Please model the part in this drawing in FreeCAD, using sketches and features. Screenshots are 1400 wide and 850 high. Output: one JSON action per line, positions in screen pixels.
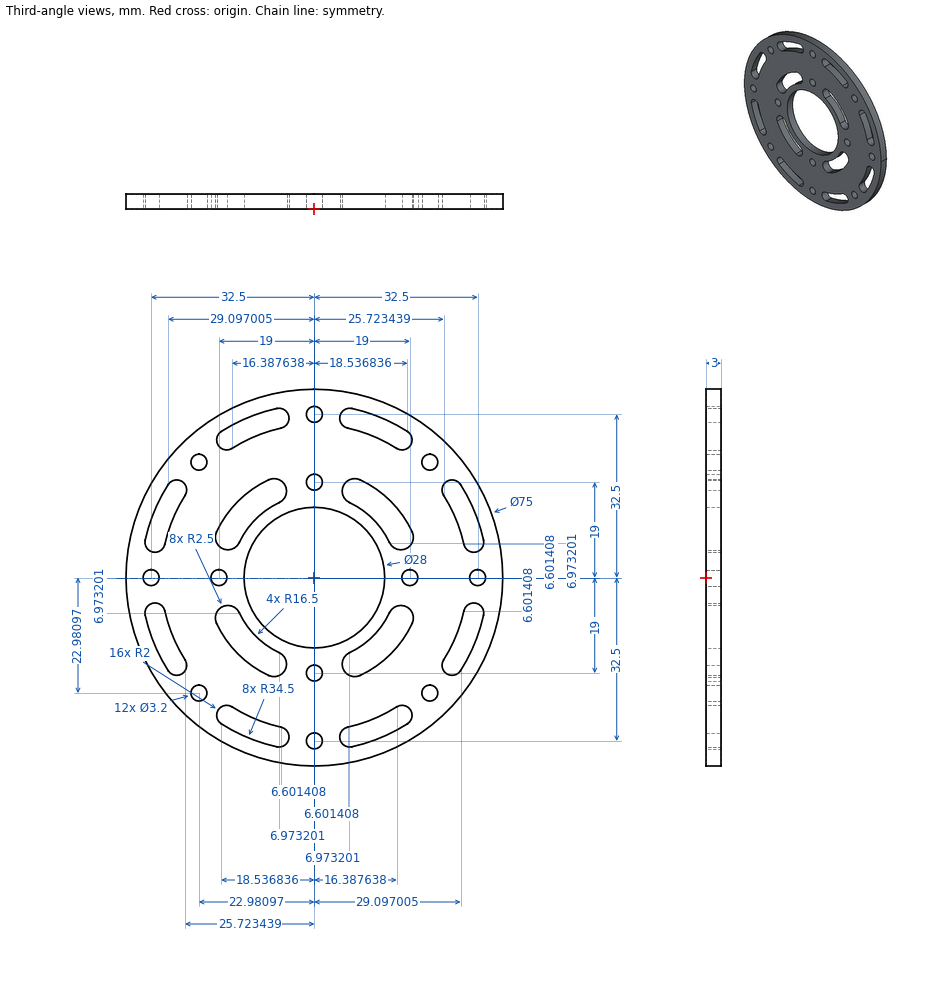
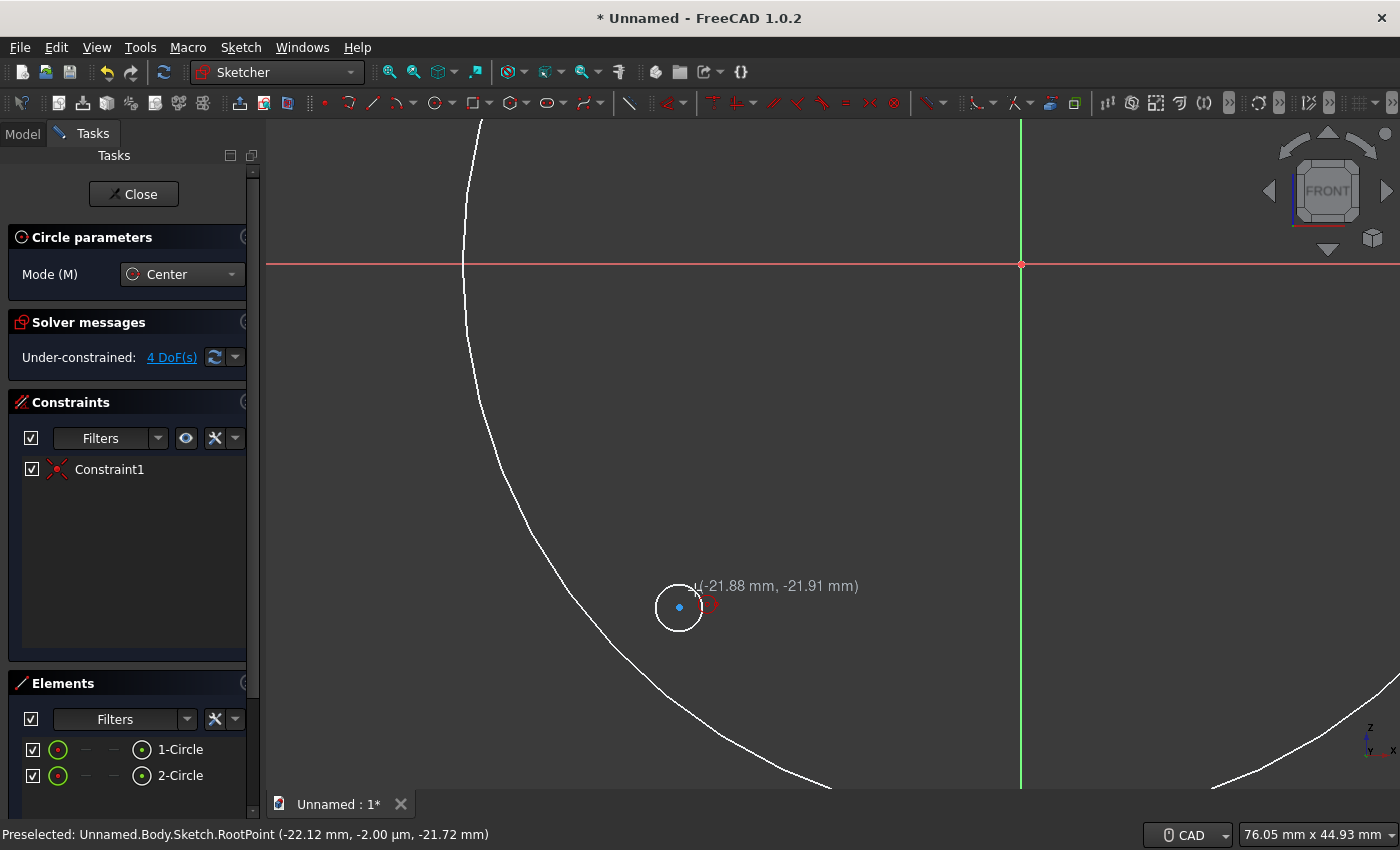
{"action": "left_click", "coordinate": [1021, 749]}
{"action": "left_click", "coordinate": [1038, 732]}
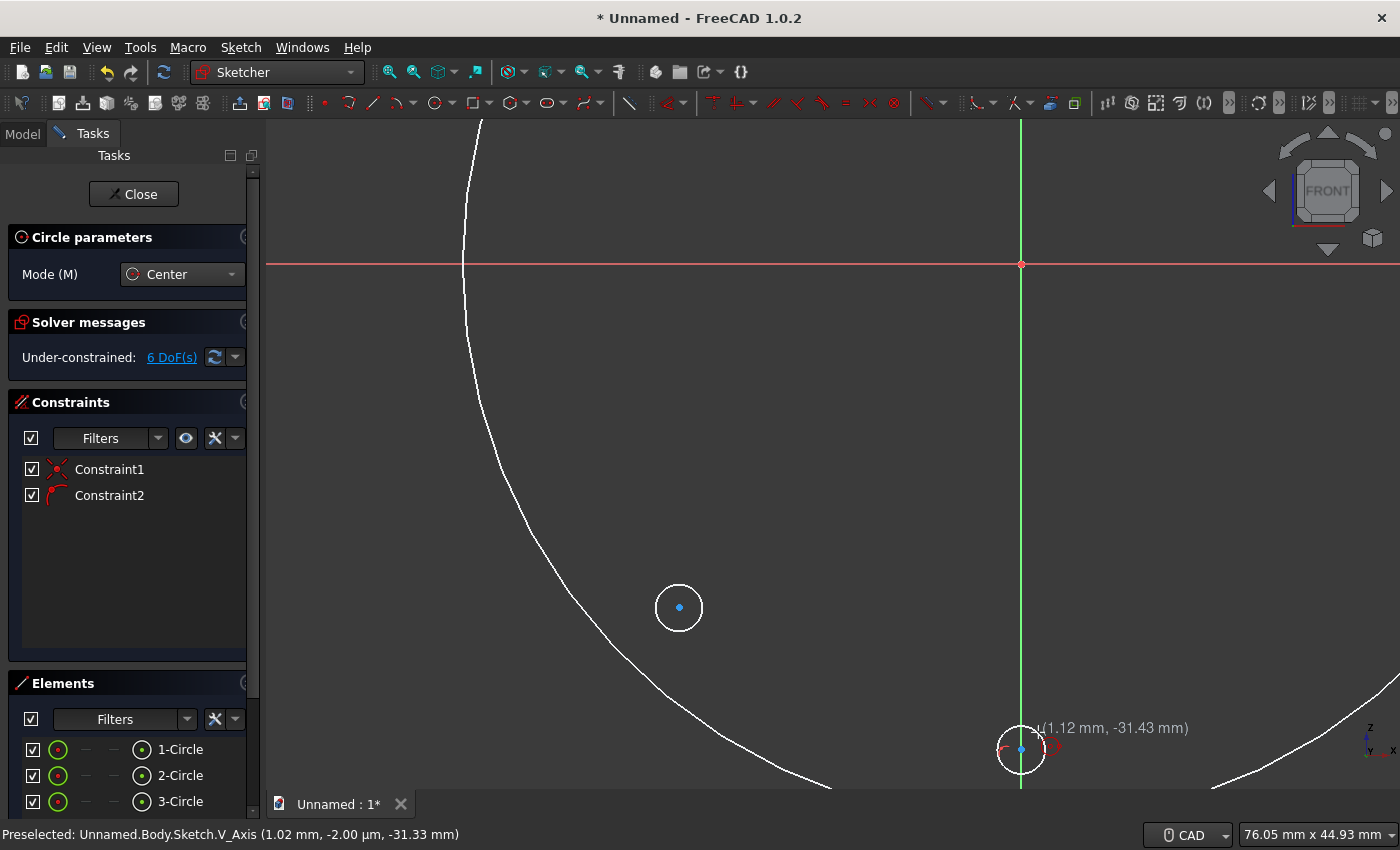
{"action": "left_click", "coordinate": [1021, 548]}
{"action": "left_click", "coordinate": [1038, 531]}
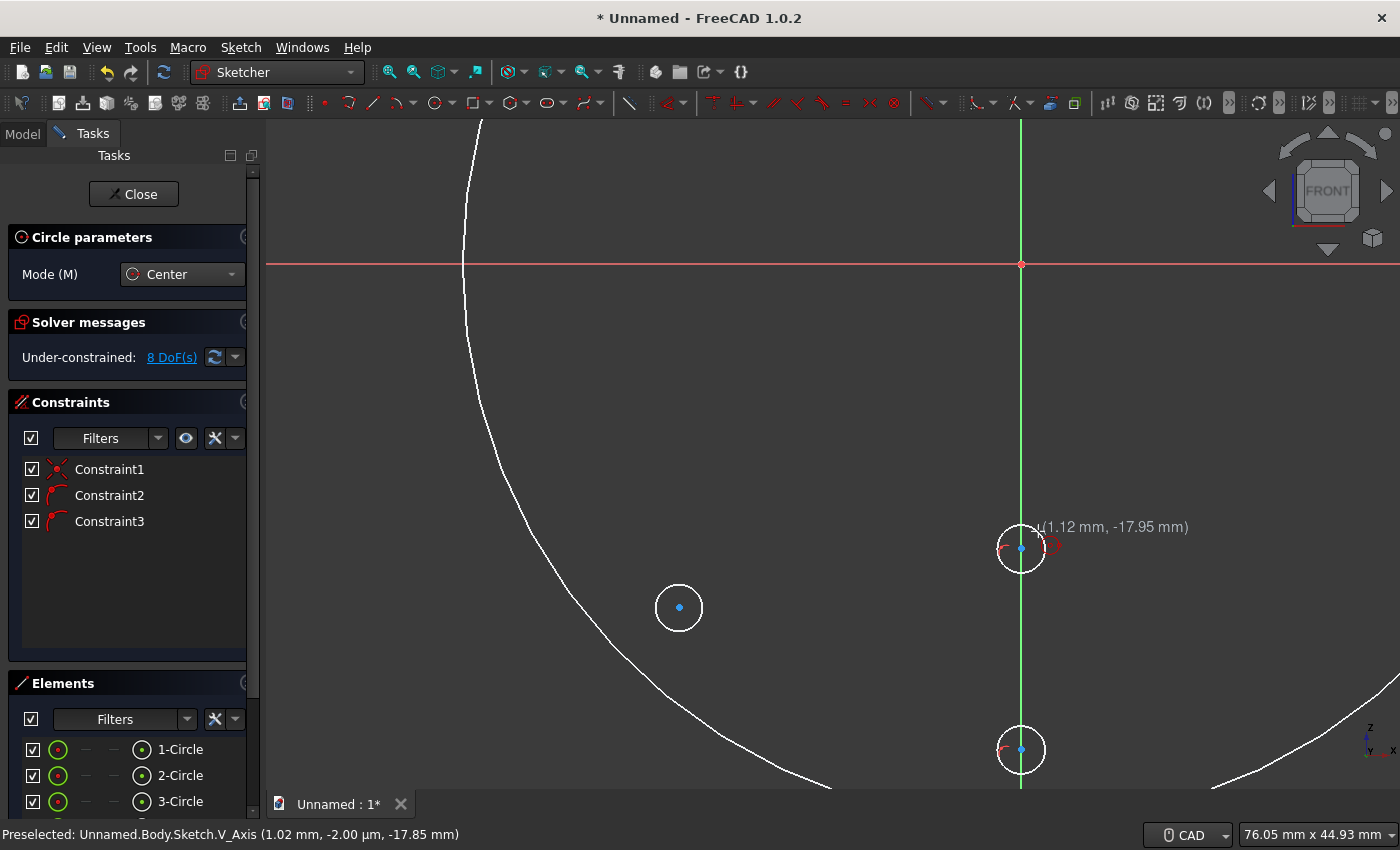
{"action": "left_click", "coordinate": [537, 264]}
{"action": "left_click", "coordinate": [554, 248]}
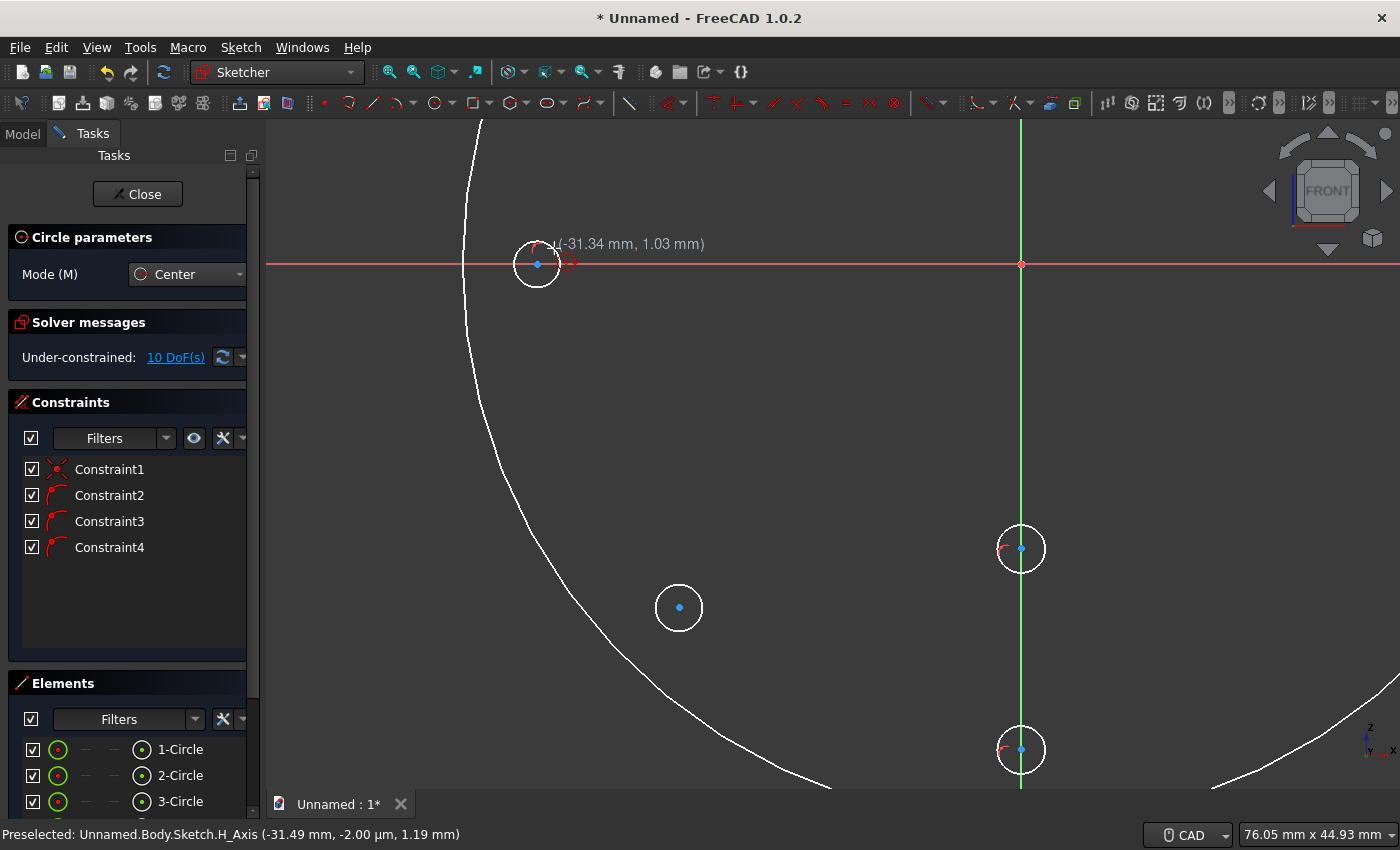
{"action": "left_click", "coordinate": [738, 264]}
{"action": "left_click", "coordinate": [755, 248]}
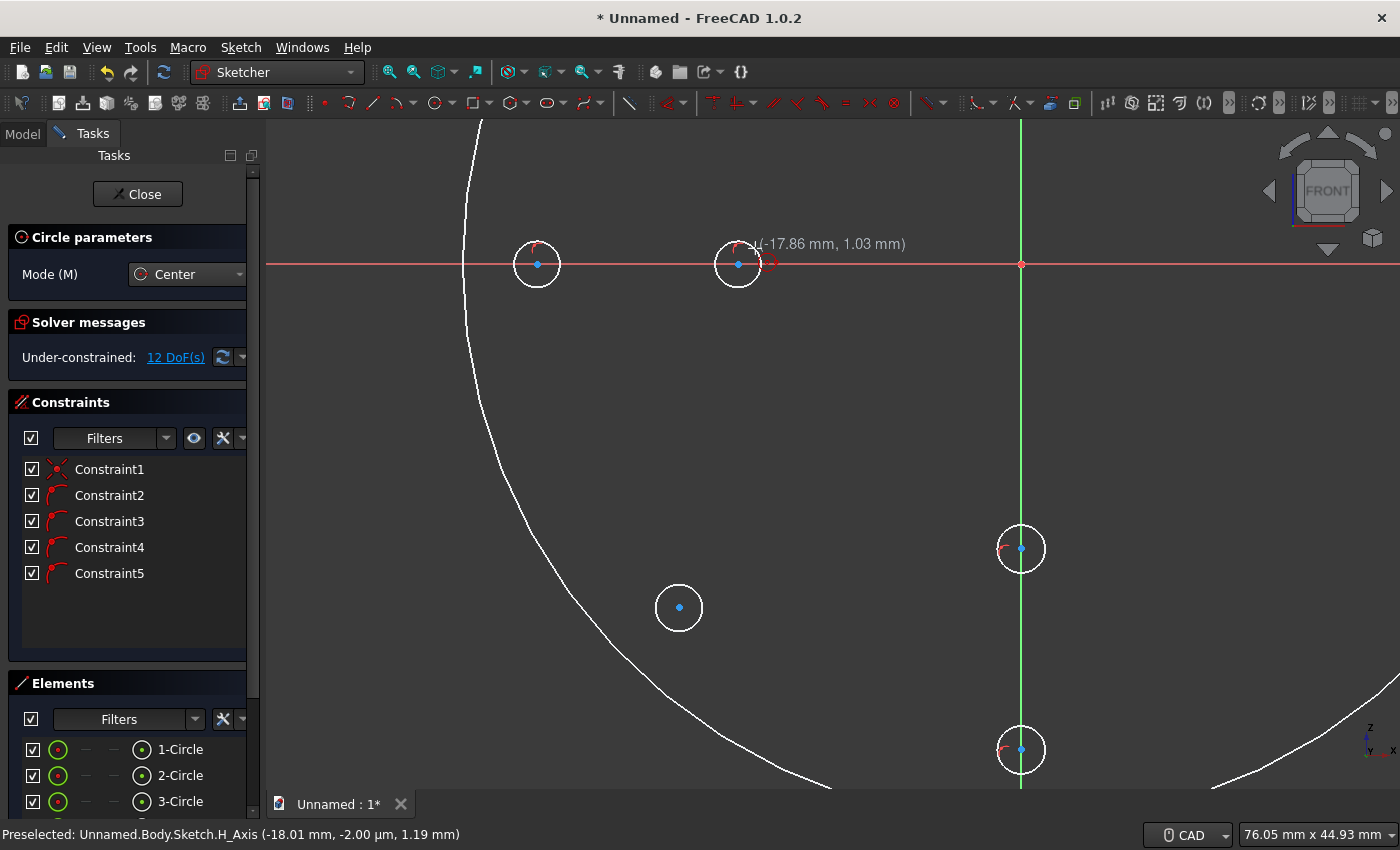
{"action": "scroll", "coordinate": [615, 564], "scroll_direction": "down", "scroll_amount": 5}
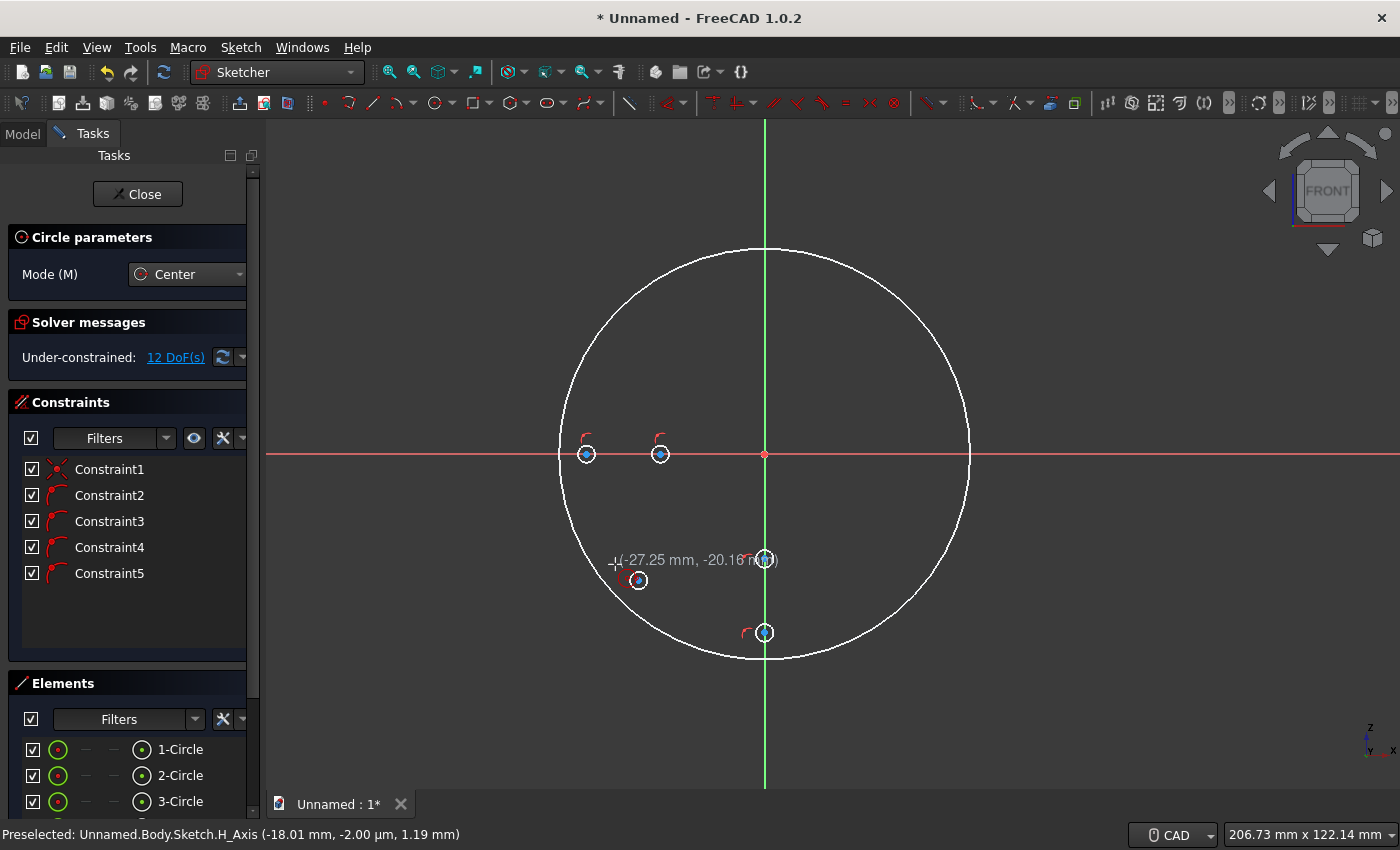
{"action": "scroll", "coordinate": [639, 328], "scroll_direction": "up", "scroll_amount": 5}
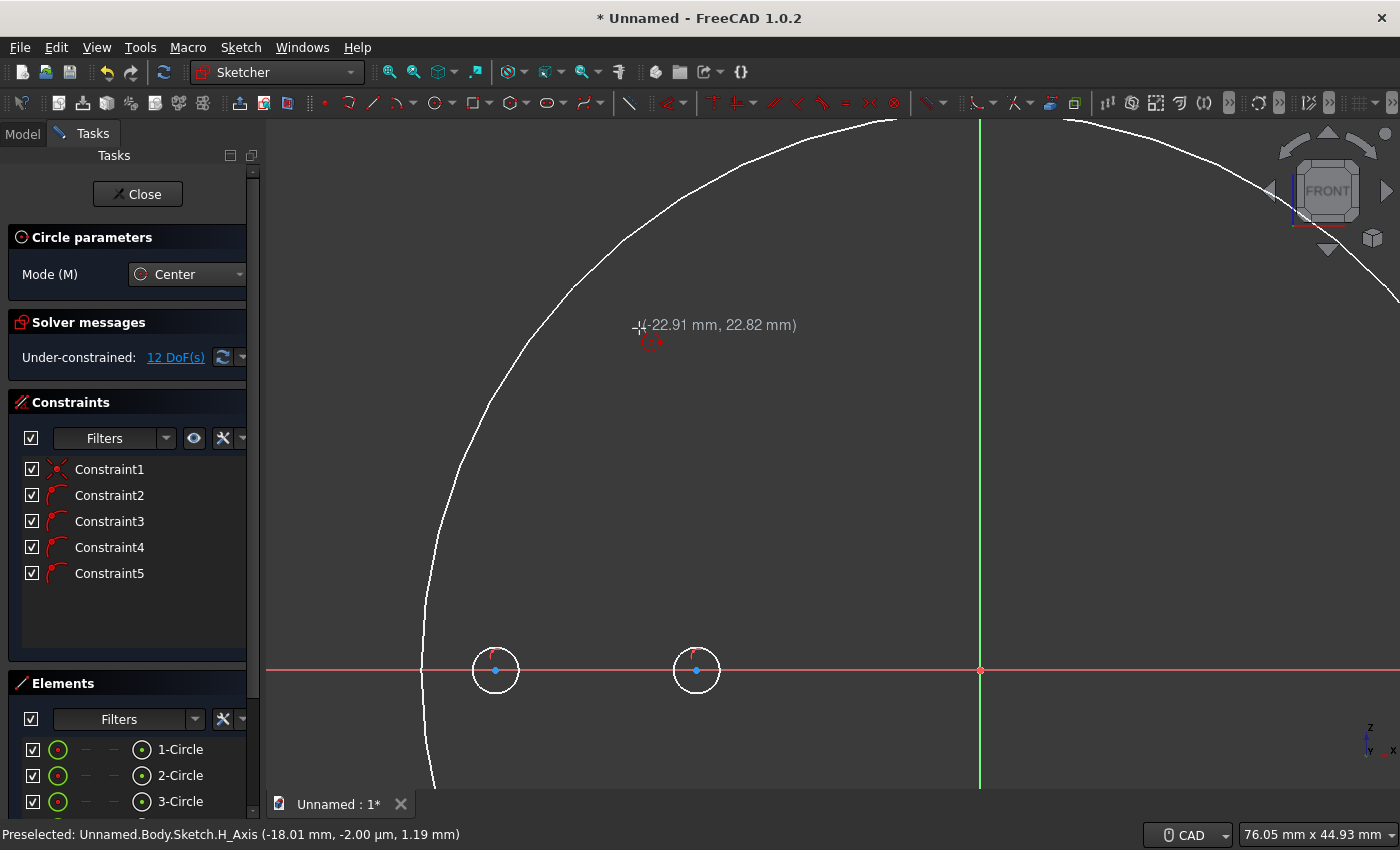
{"action": "left_click", "coordinate": [637, 328]}
{"action": "left_click", "coordinate": [654, 311]}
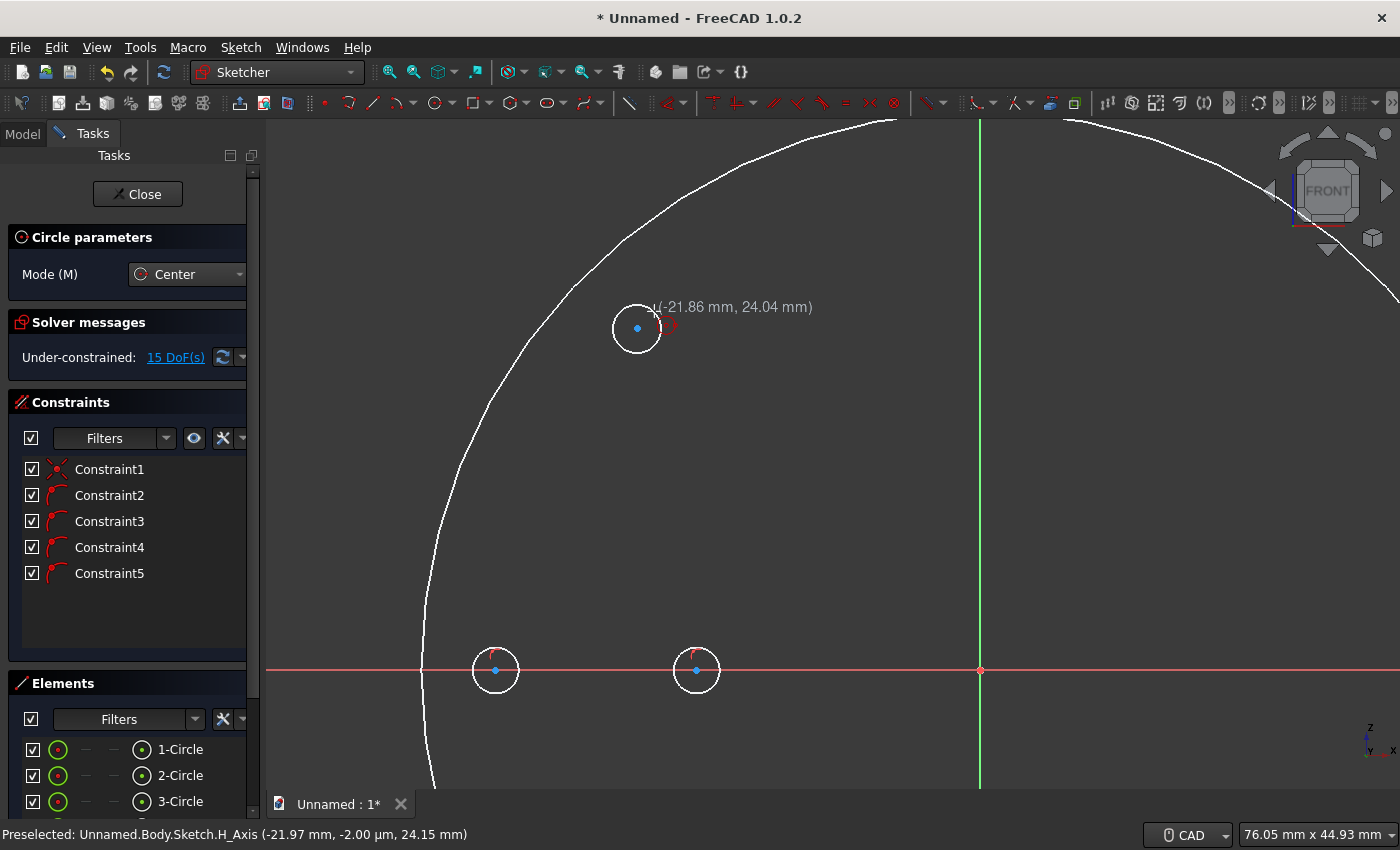
{"action": "scroll", "coordinate": [639, 328], "scroll_direction": "down", "scroll_amount": 5}